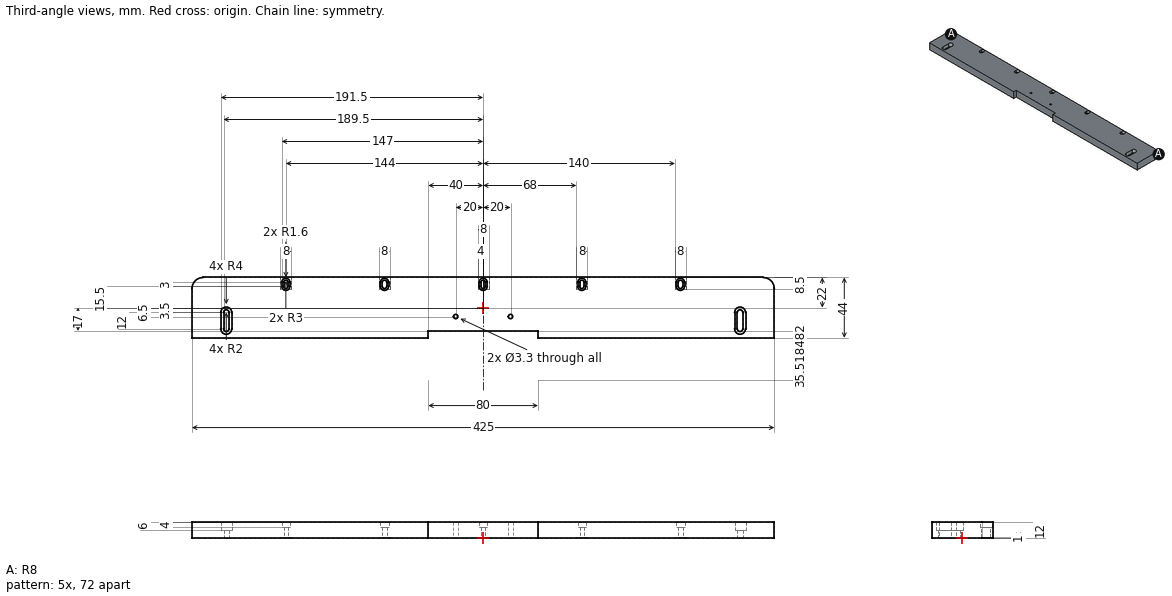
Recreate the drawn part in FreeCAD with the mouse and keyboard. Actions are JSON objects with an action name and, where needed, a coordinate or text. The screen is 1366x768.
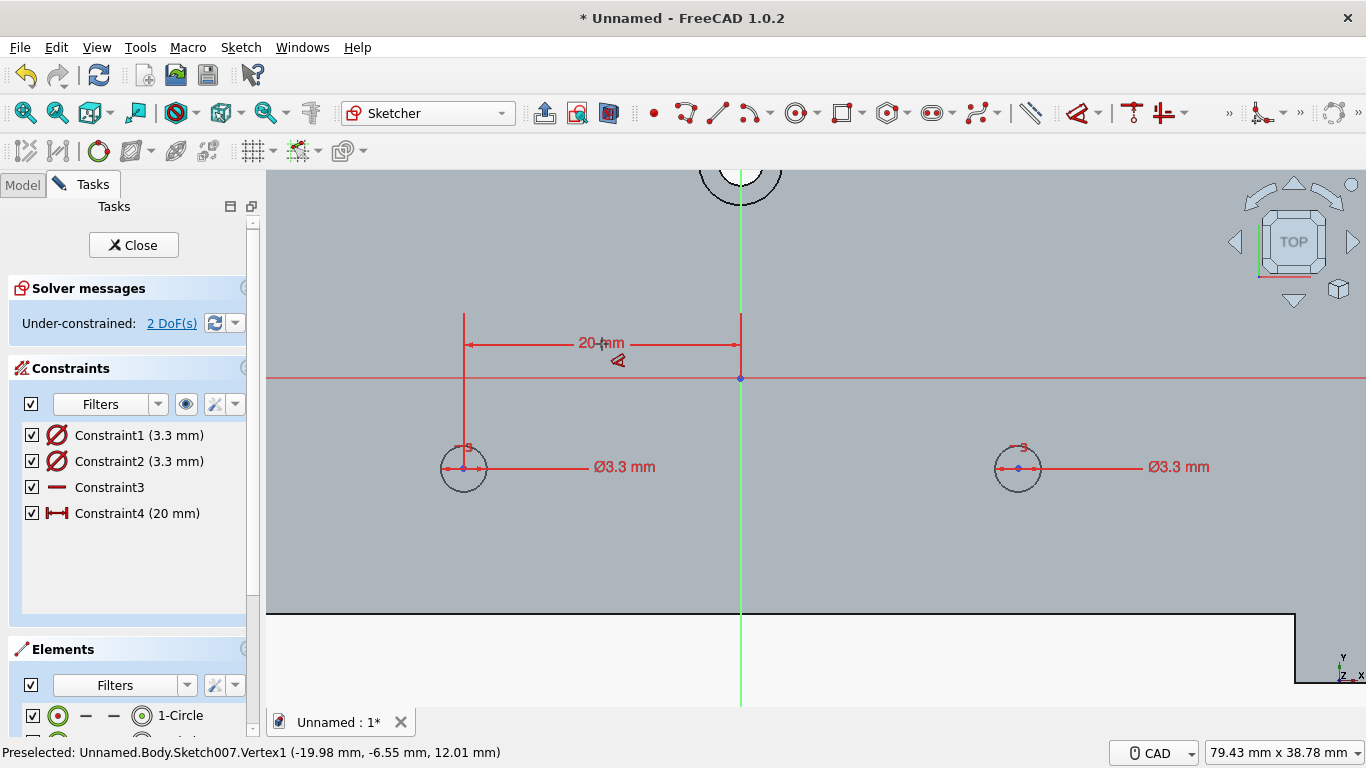
{"action": "left_click", "coordinate": [1018, 469]}
{"action": "left_click", "coordinate": [879, 344]}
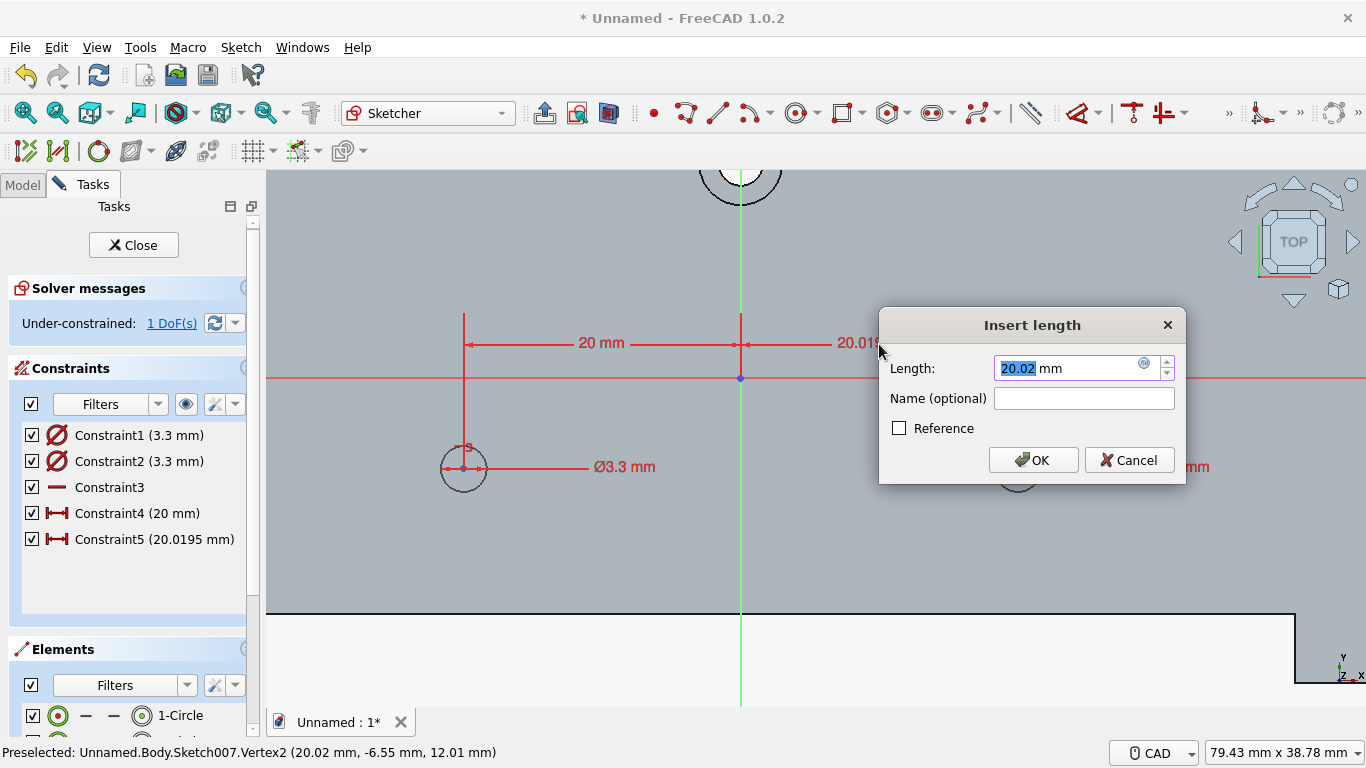
{"action": "type", "text": "20"}
{"action": "key", "text": "Return"}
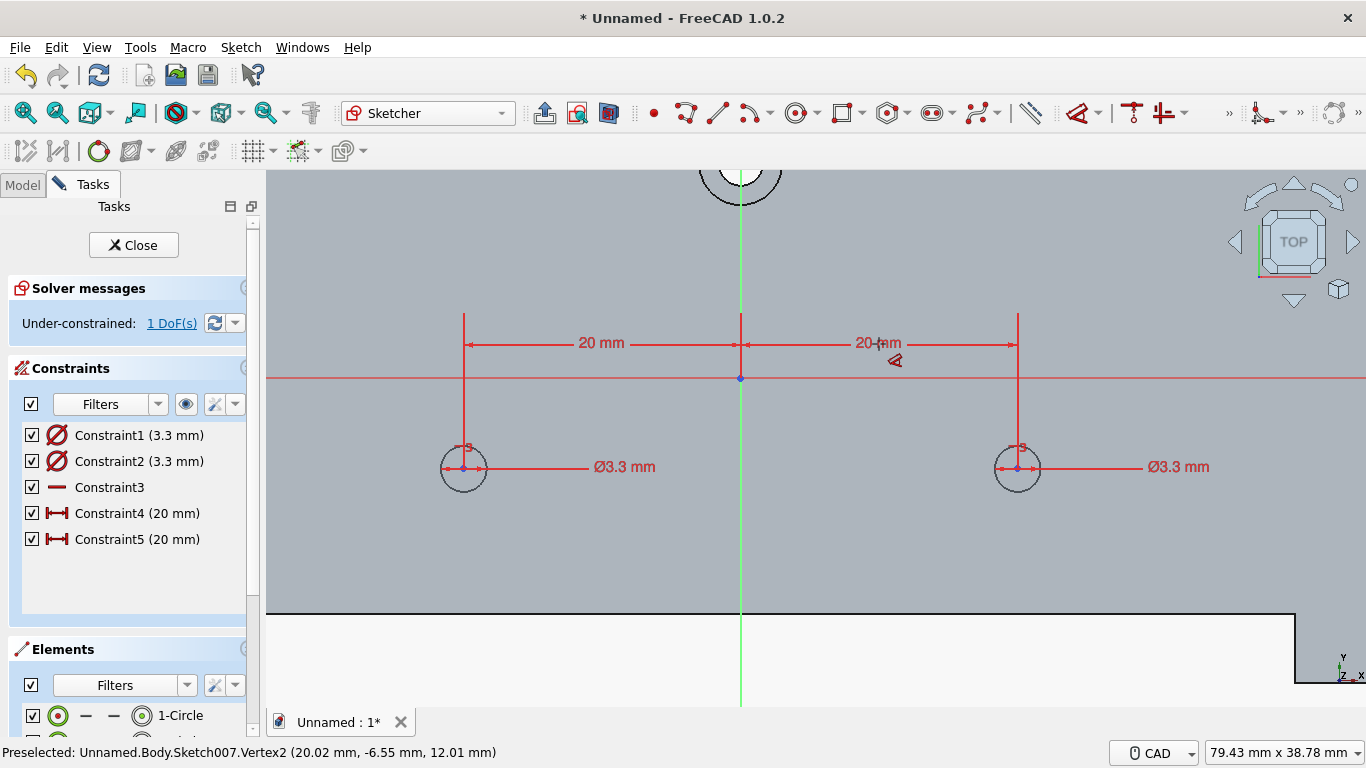
{"action": "left_click", "coordinate": [464, 469]}
{"action": "left_click", "coordinate": [430, 424]}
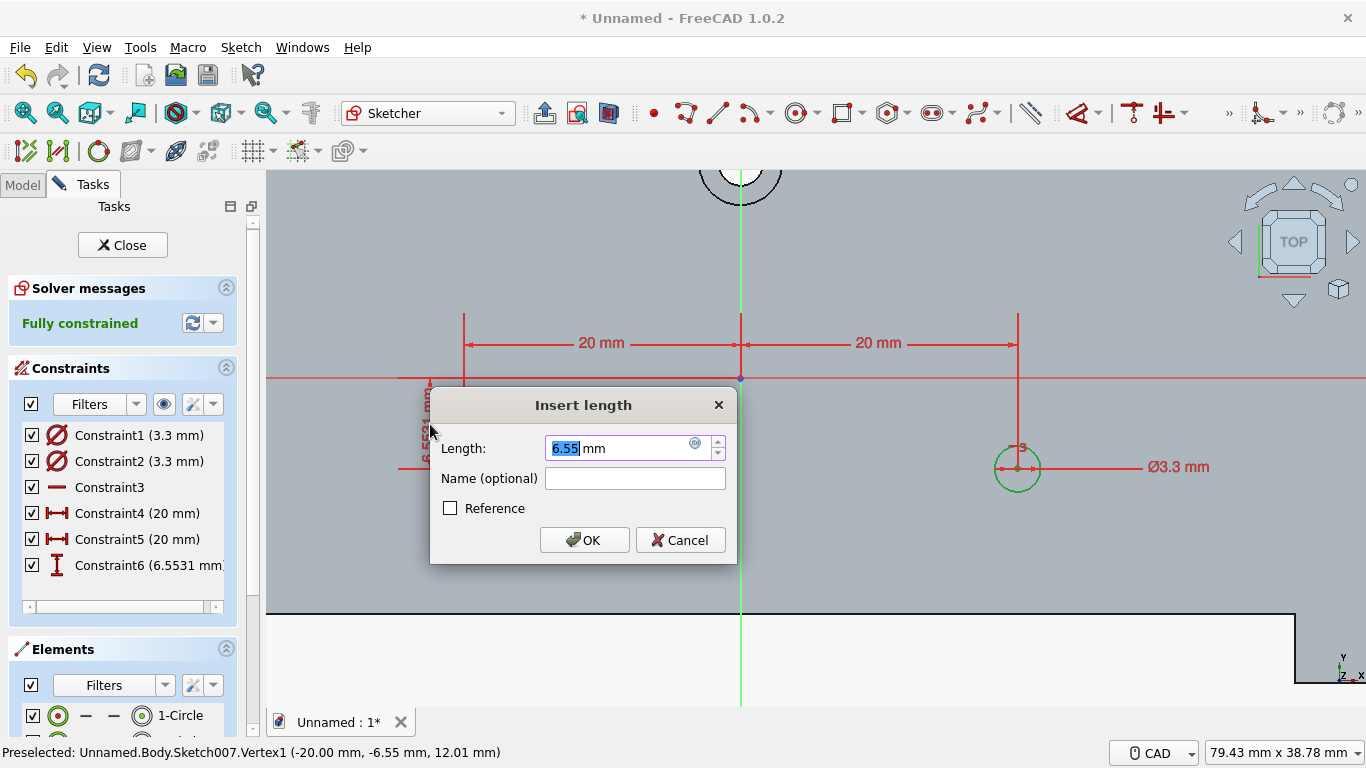
{"action": "type", "text": "6.5"}
{"action": "key", "text": "Return"}
{"action": "key", "text": "Escape"}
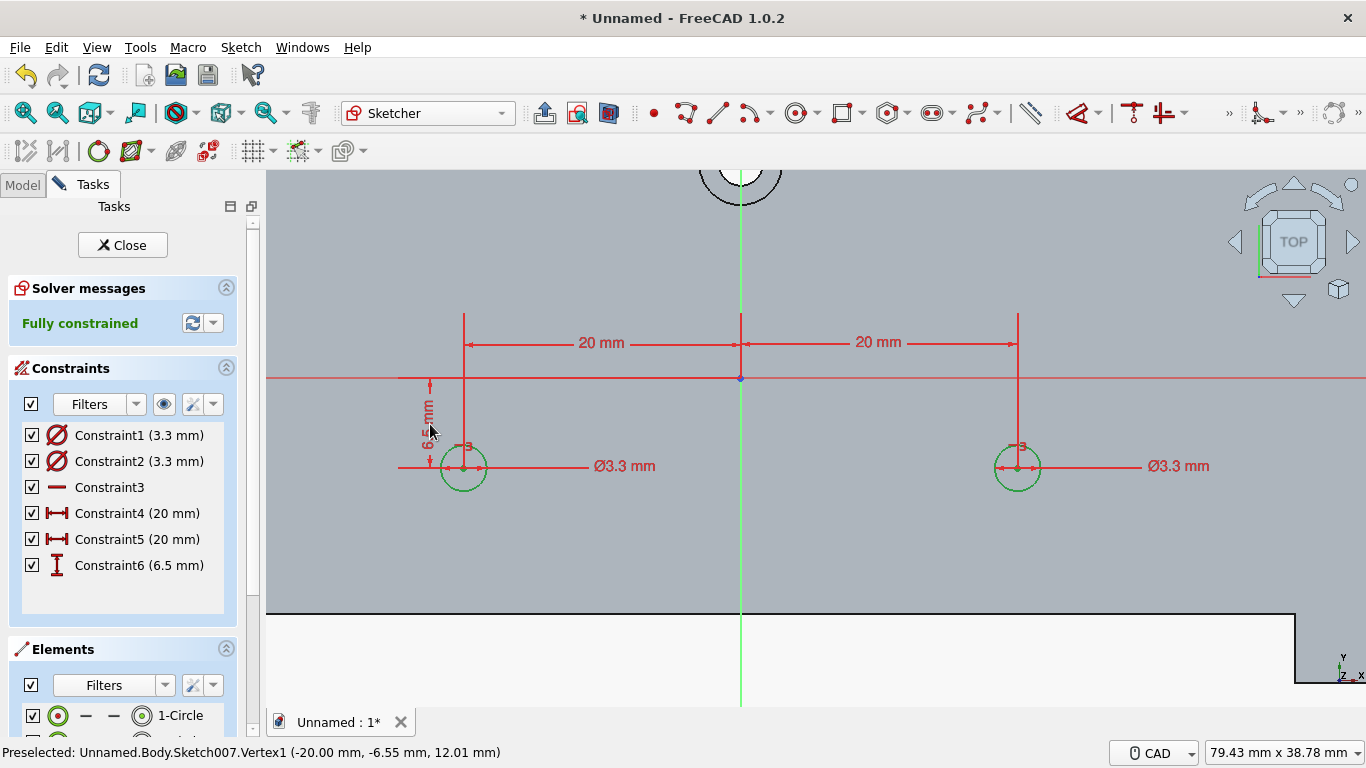
{"action": "left_click", "coordinate": [123, 245]}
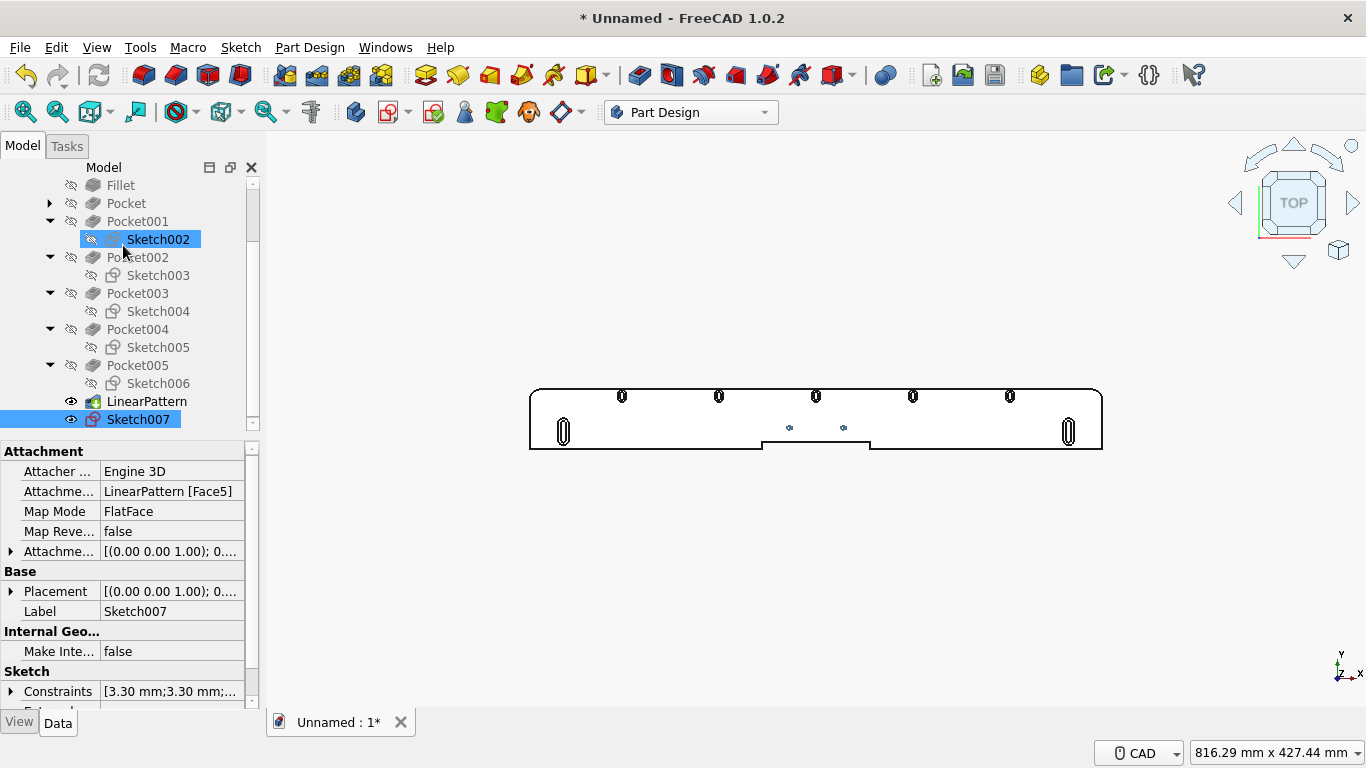
{"action": "left_click", "coordinate": [672, 76]}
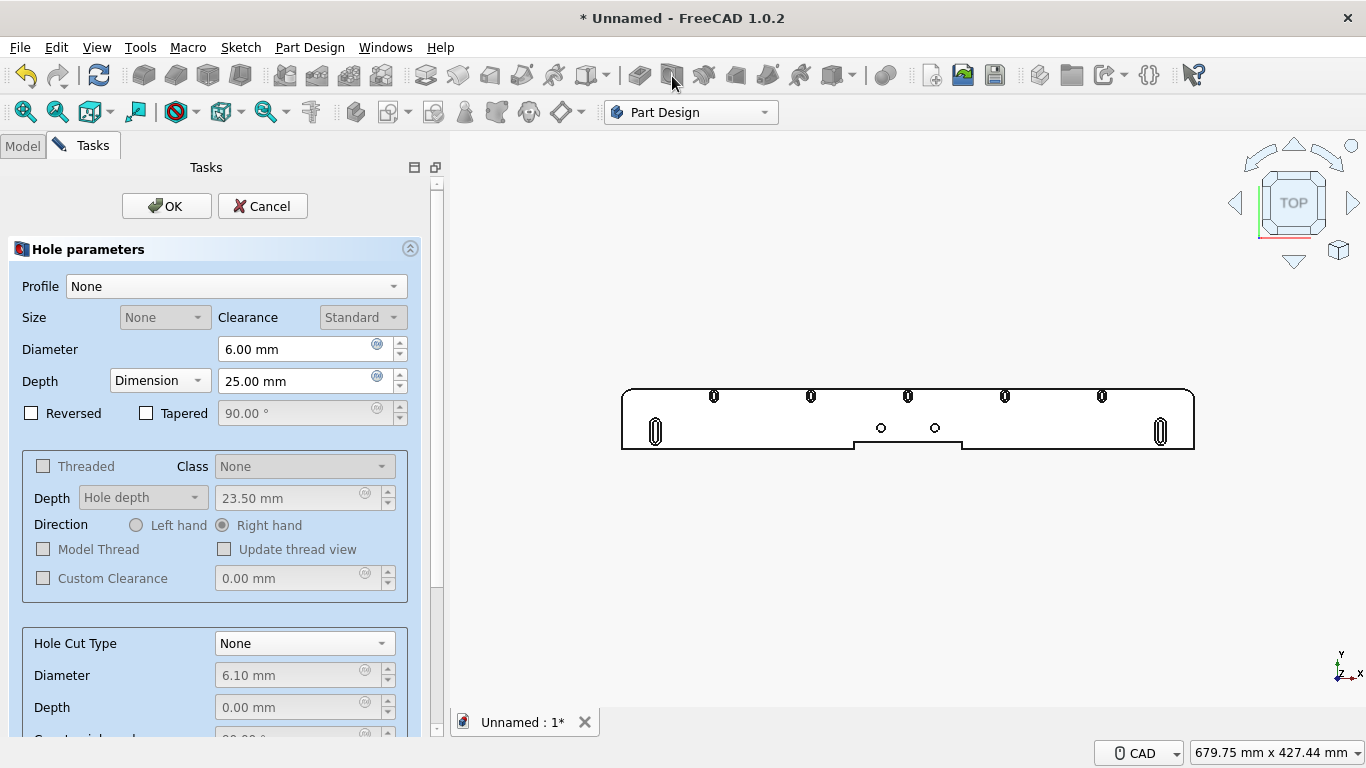
{"action": "triple_click", "coordinate": [305, 349]}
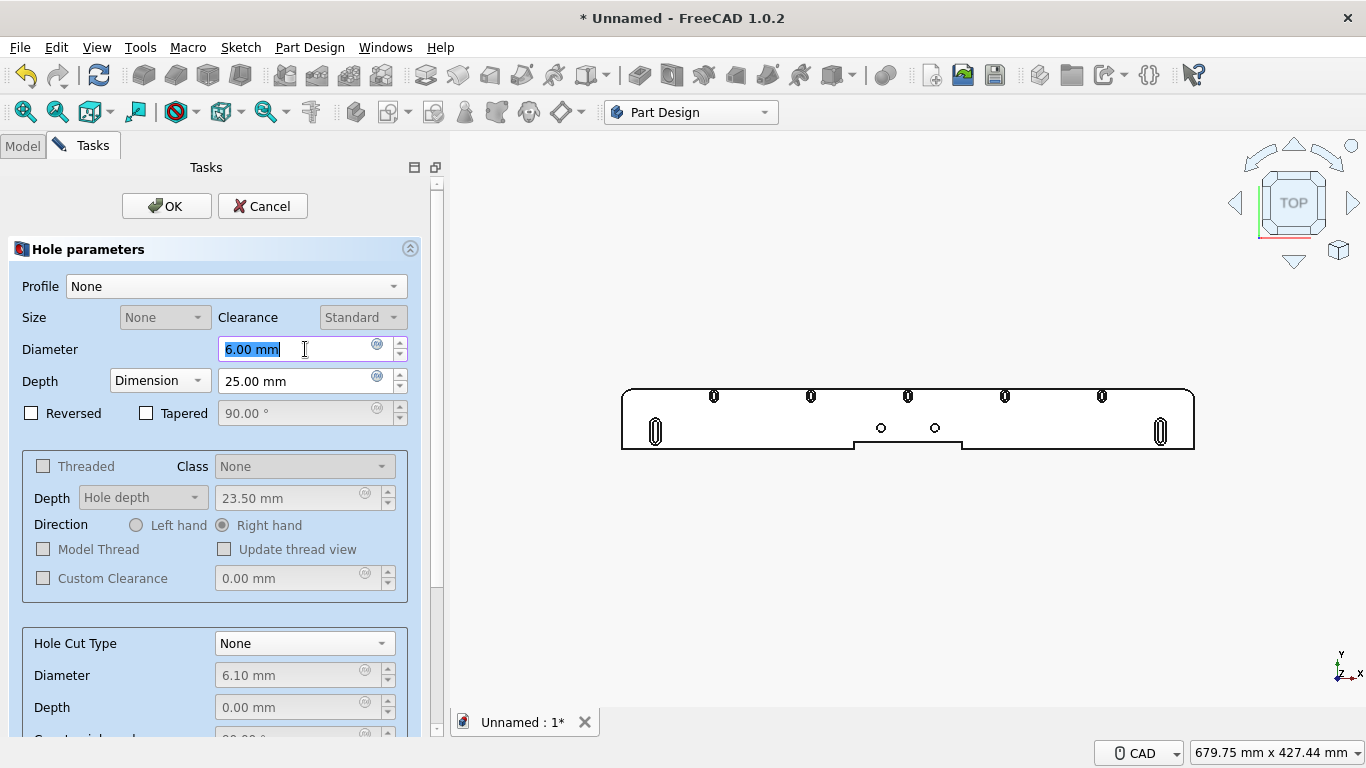
{"action": "type", "text": "3.3"}
{"action": "key", "text": "Tab"}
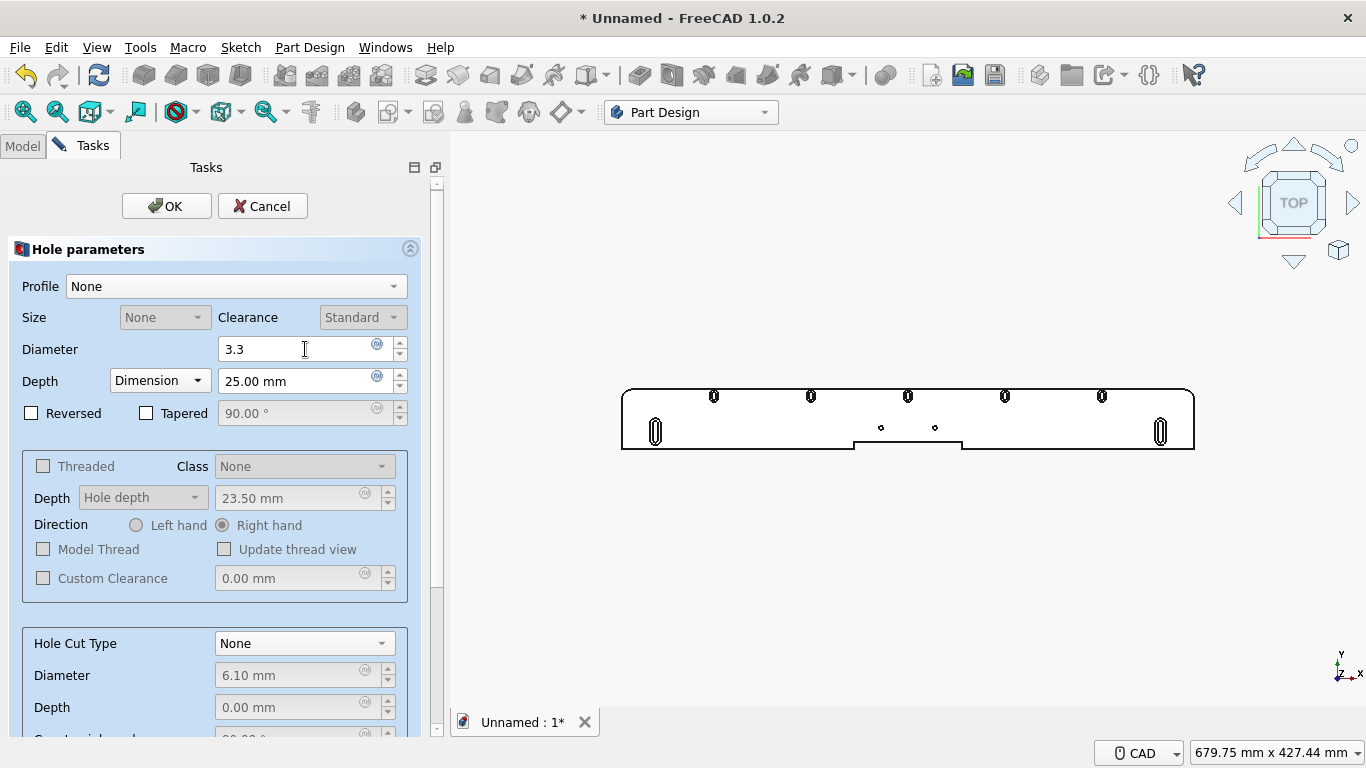
{"action": "left_click", "coordinate": [161, 380]}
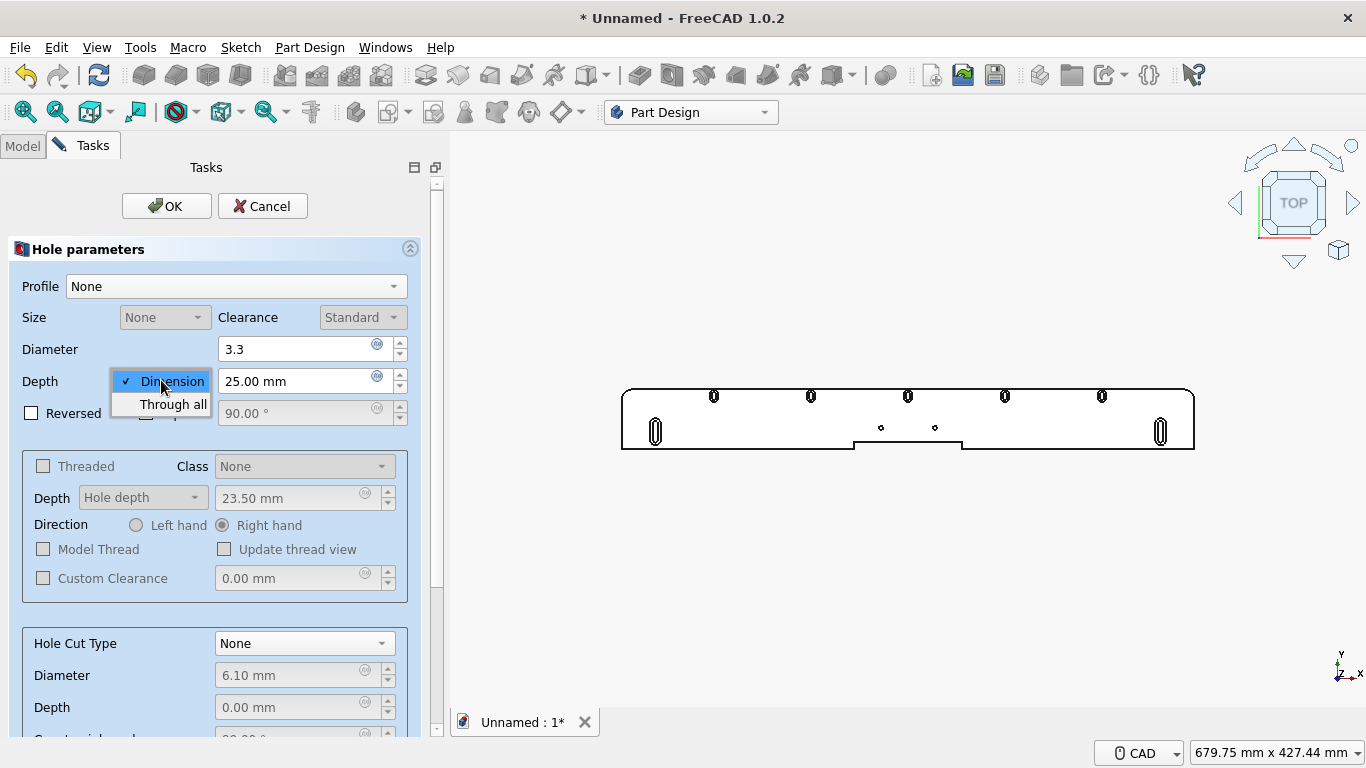
{"action": "left_click", "coordinate": [160, 404]}